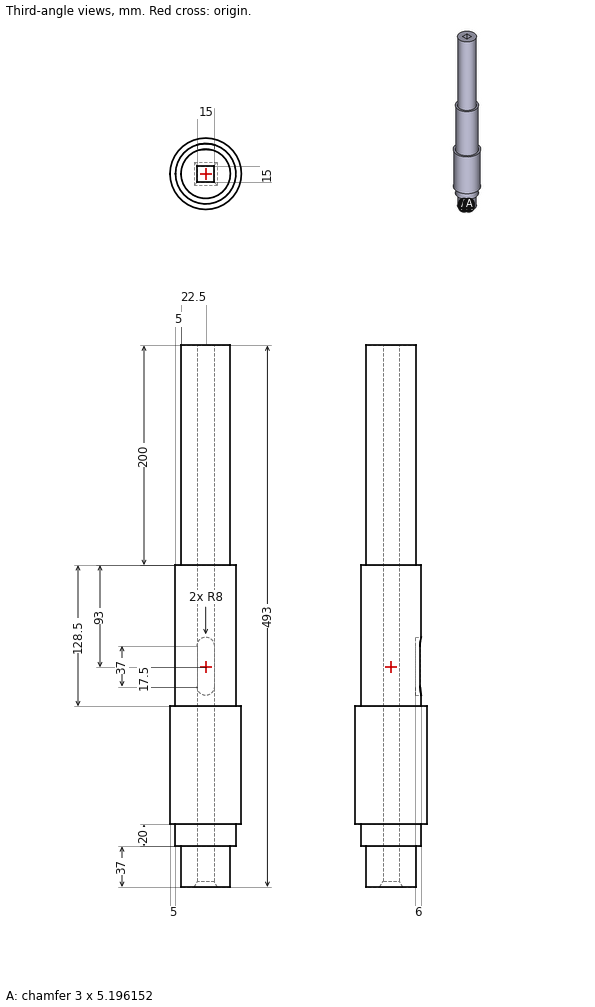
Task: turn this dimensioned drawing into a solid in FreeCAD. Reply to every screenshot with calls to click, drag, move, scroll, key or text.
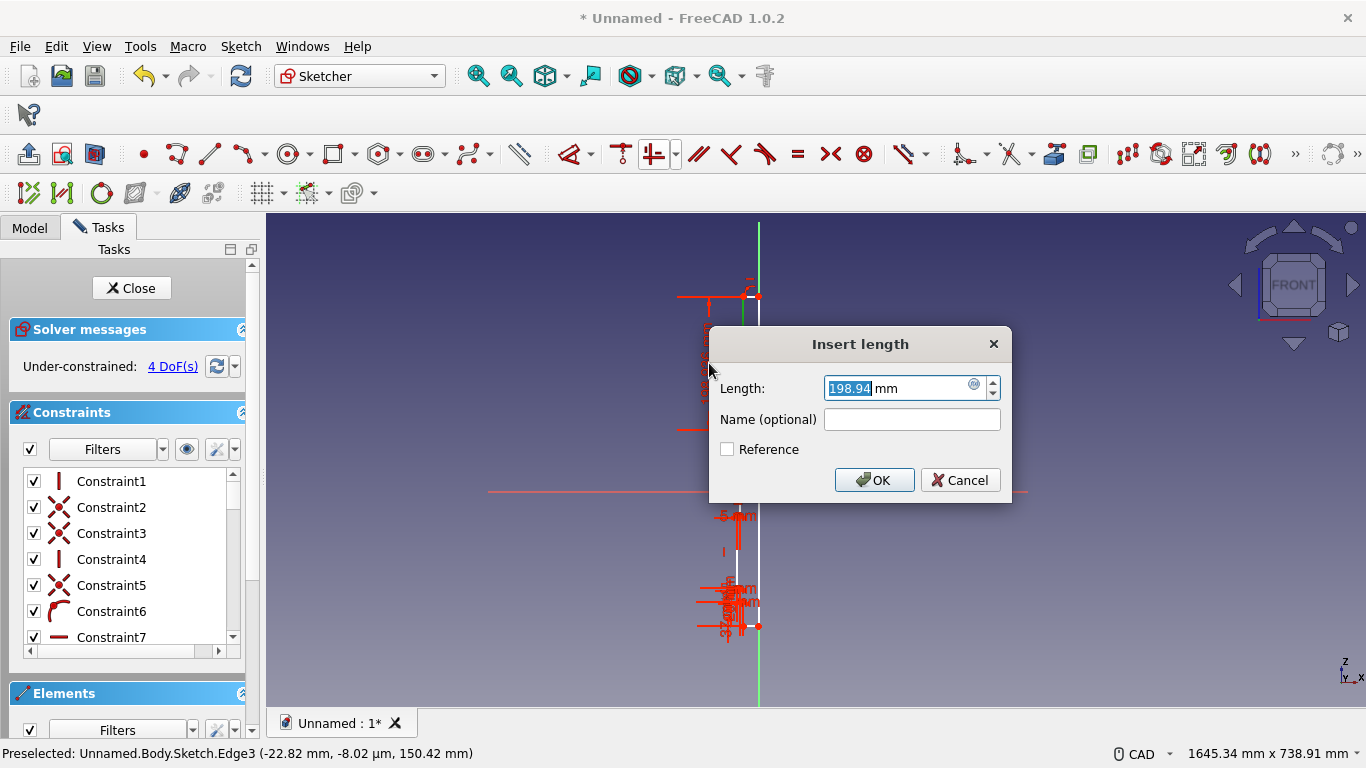
text(200)
key(Return)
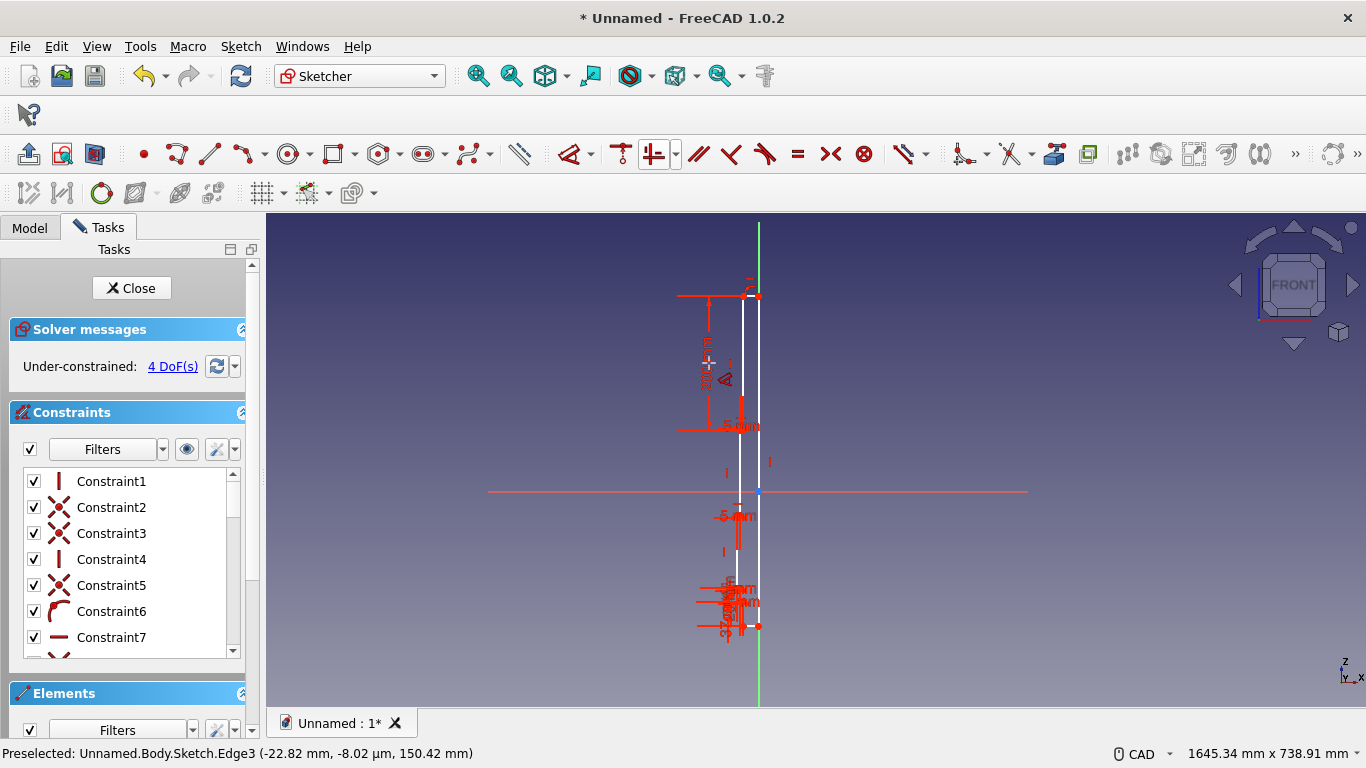
click(759, 395)
click(793, 461)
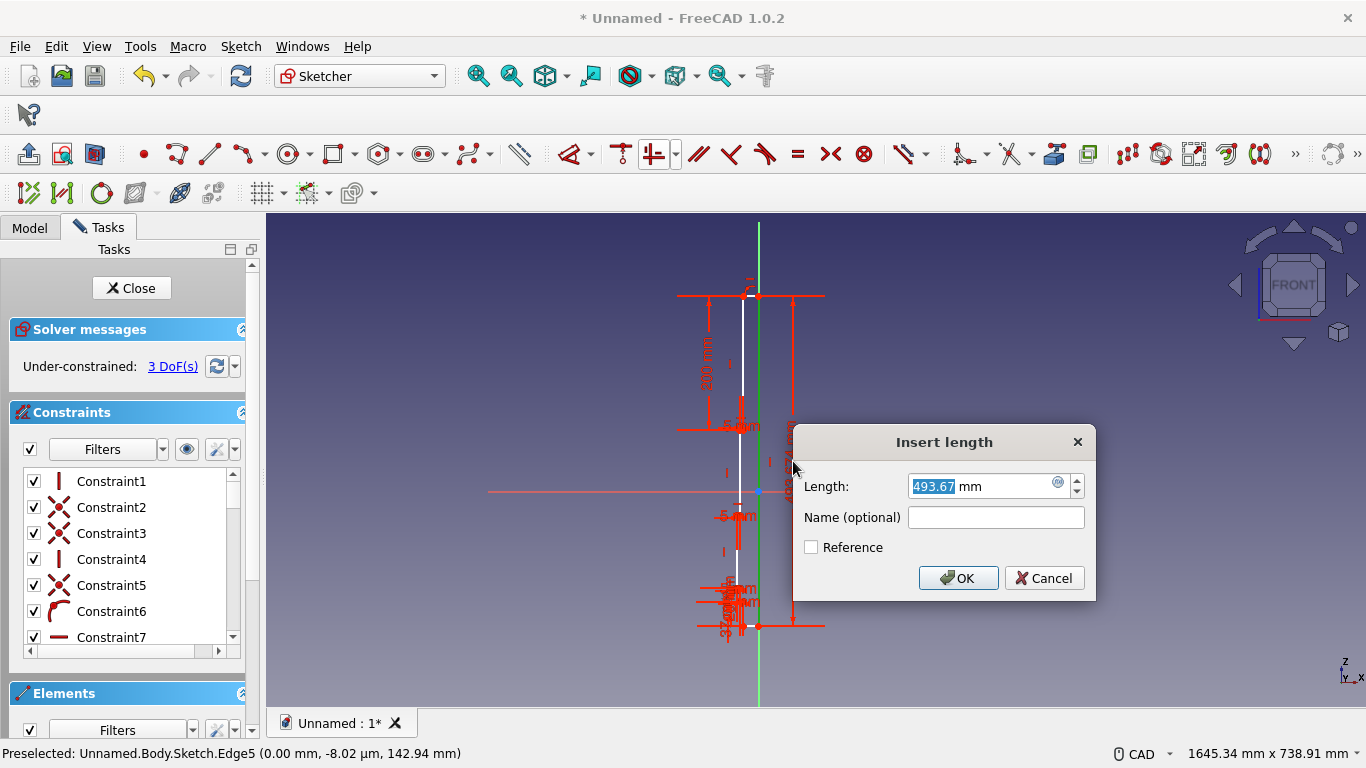
text(493)
key(Return)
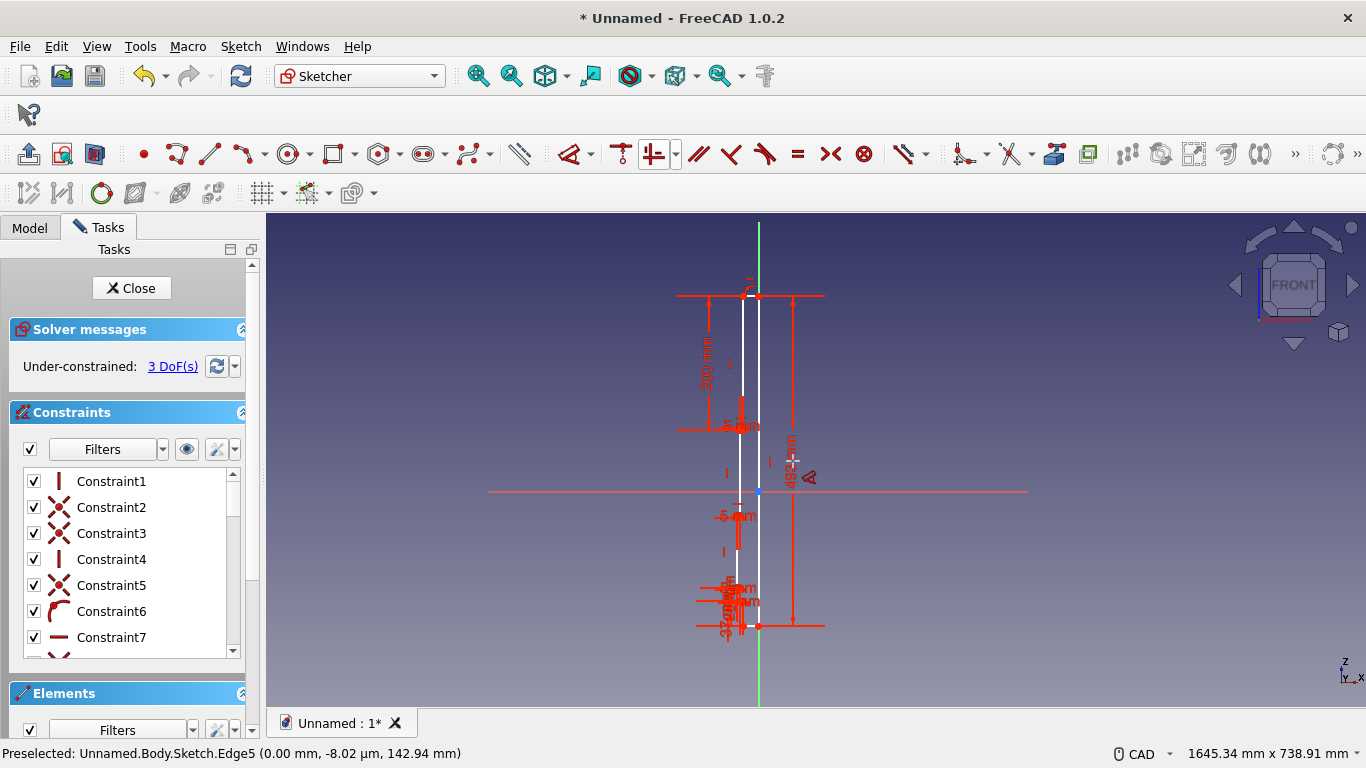
scroll(740, 430, up, 7)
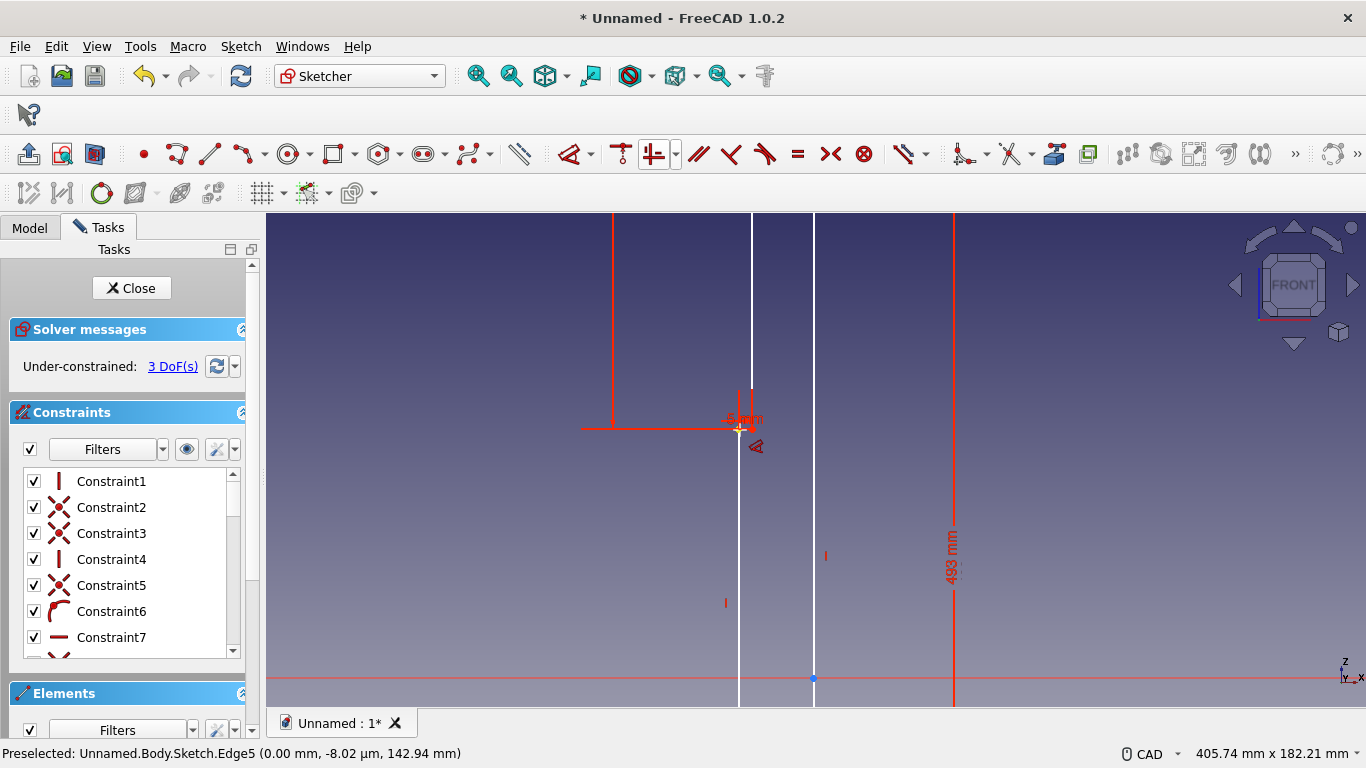
click(739, 429)
click(848, 554)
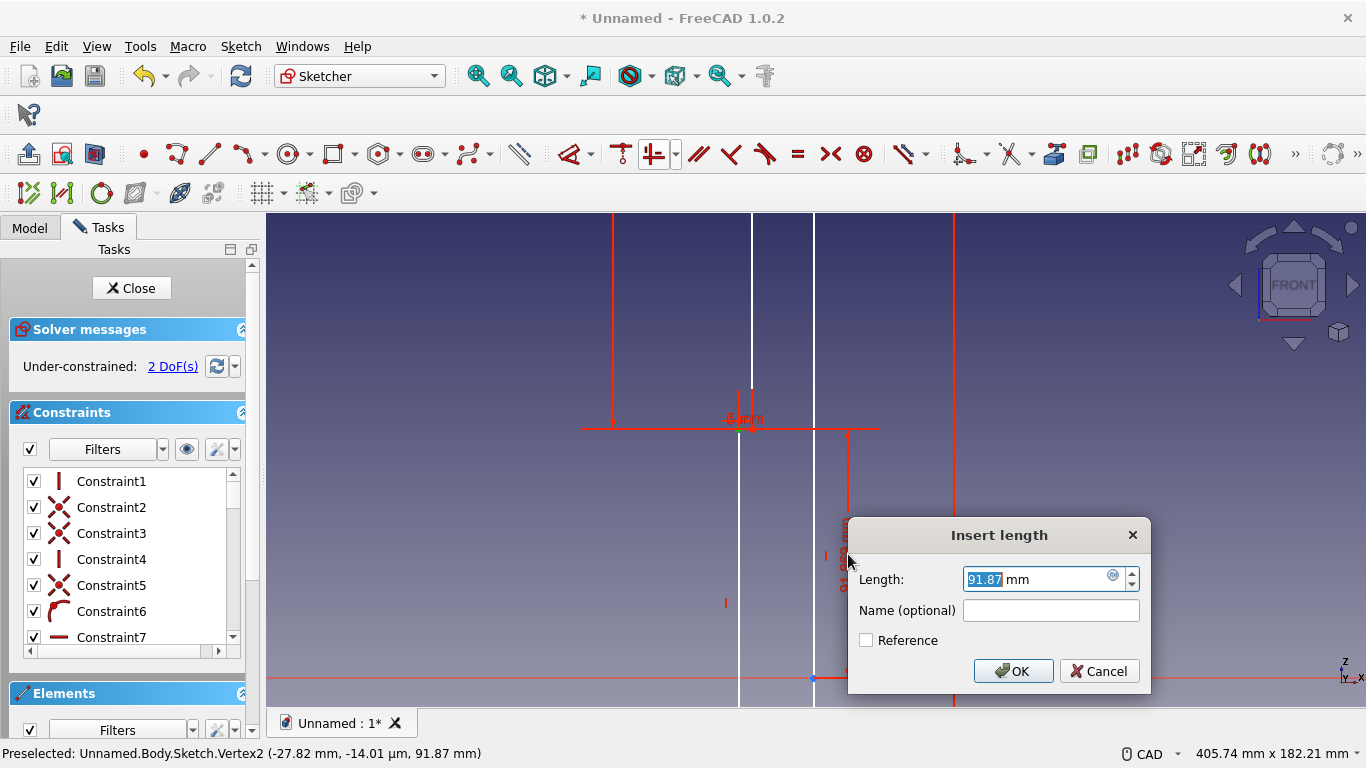
text(93)
key(Return)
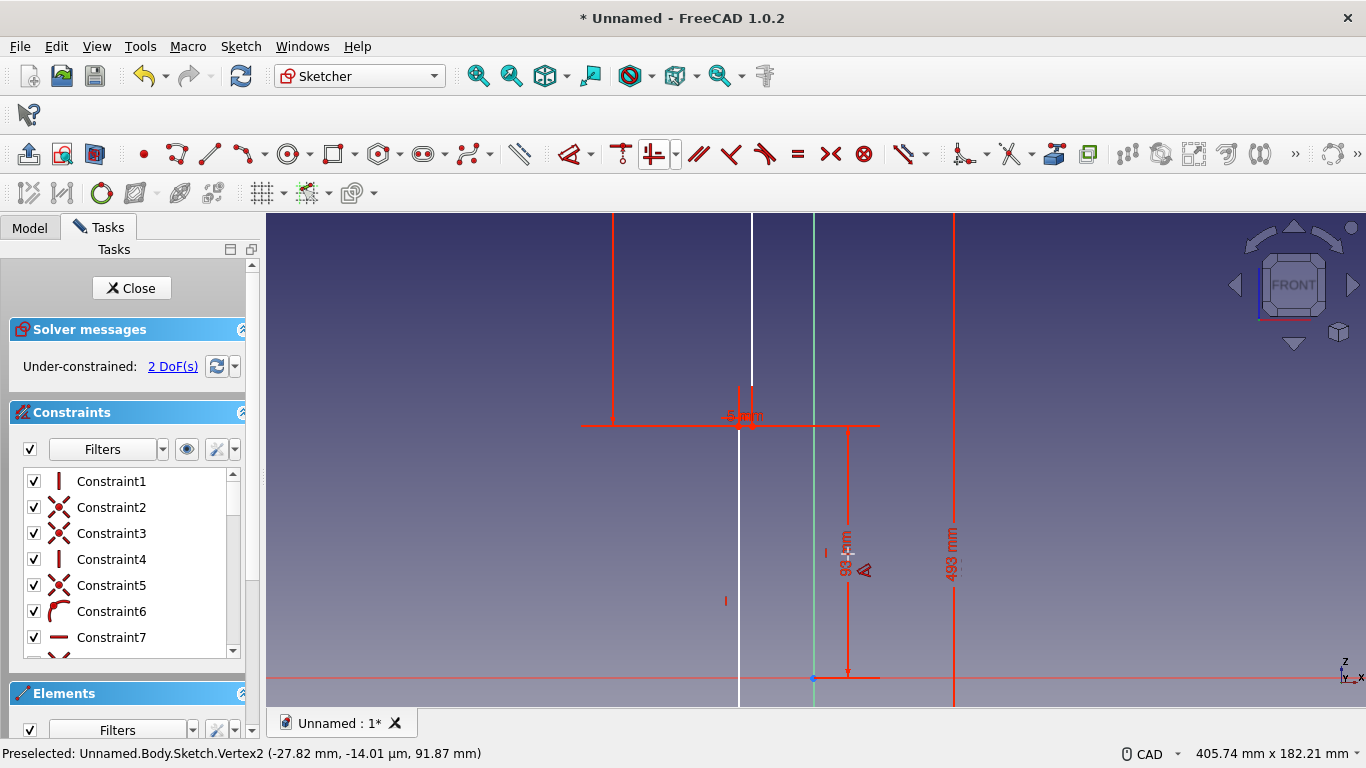
scroll(740, 430, down, 7)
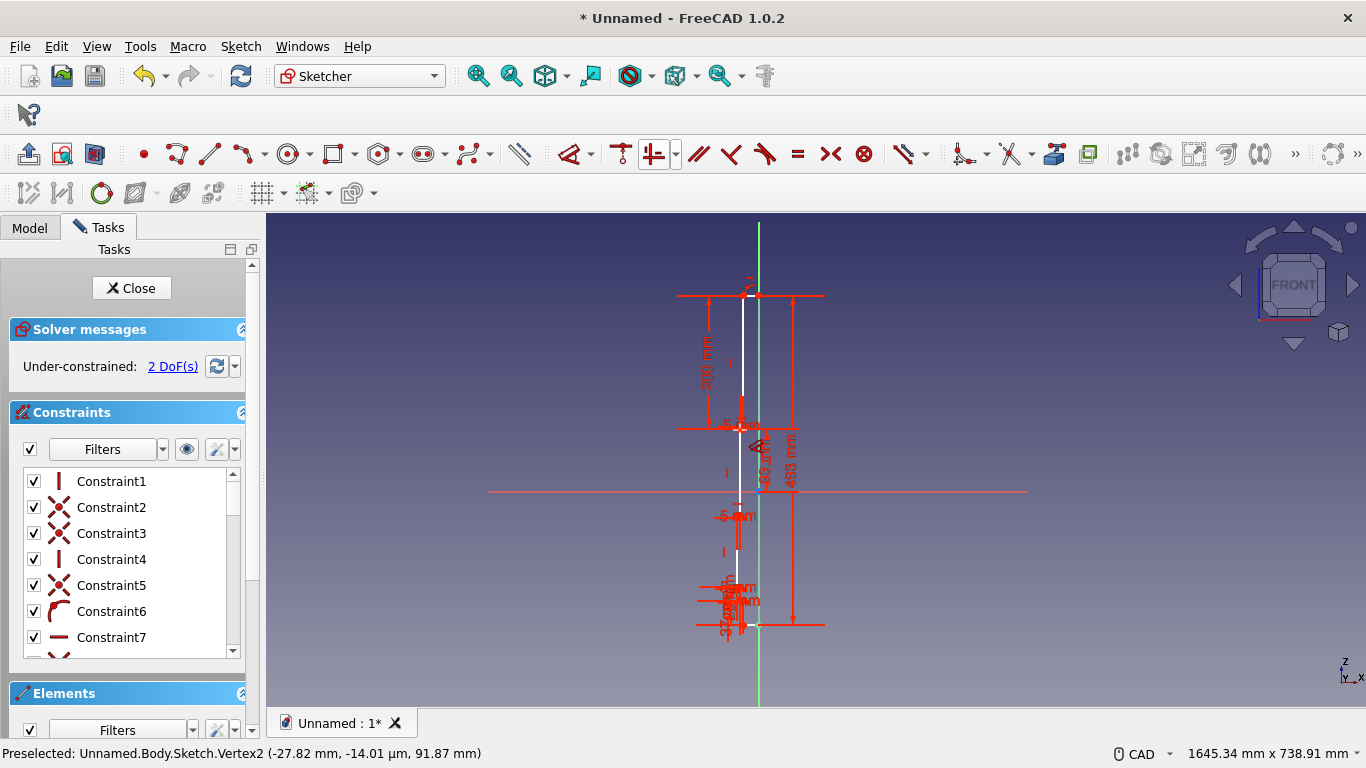
scroll(748, 296, up, 6)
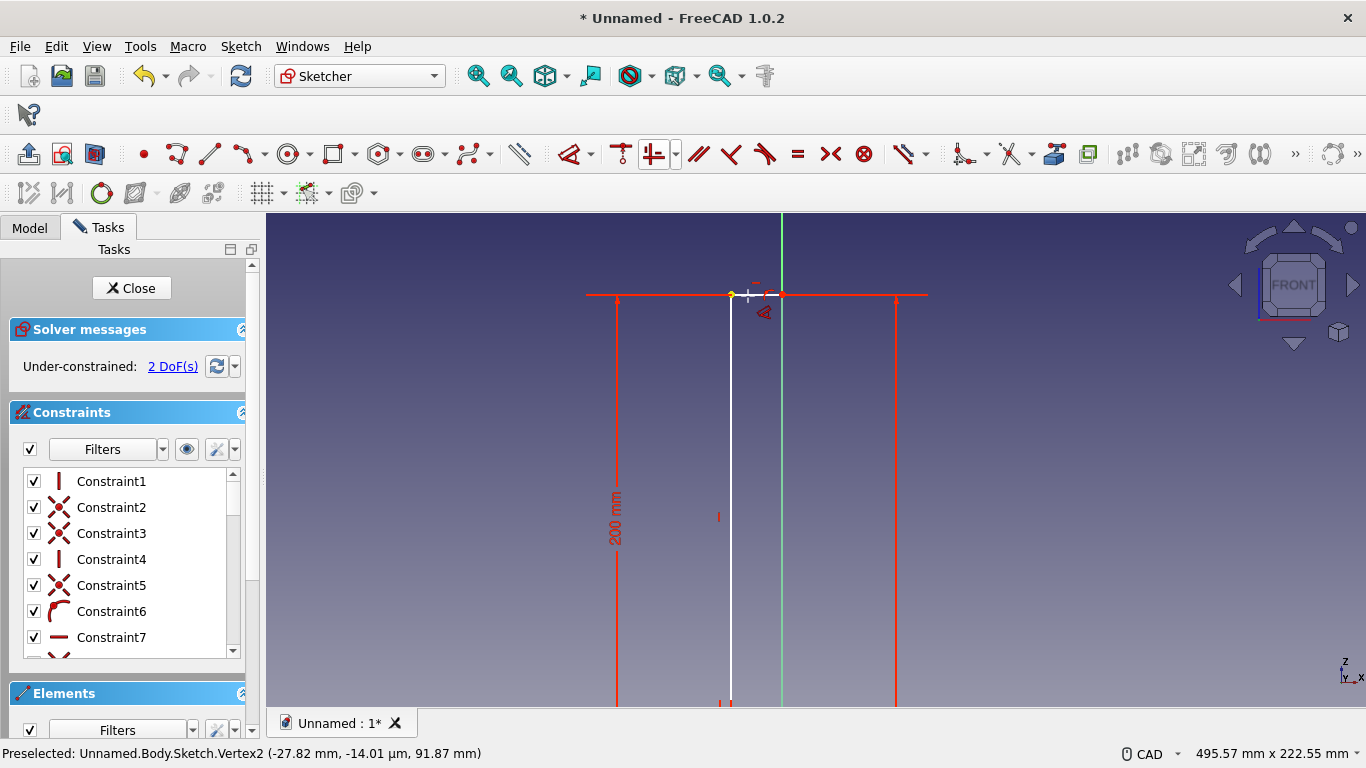
click(747, 295)
click(757, 261)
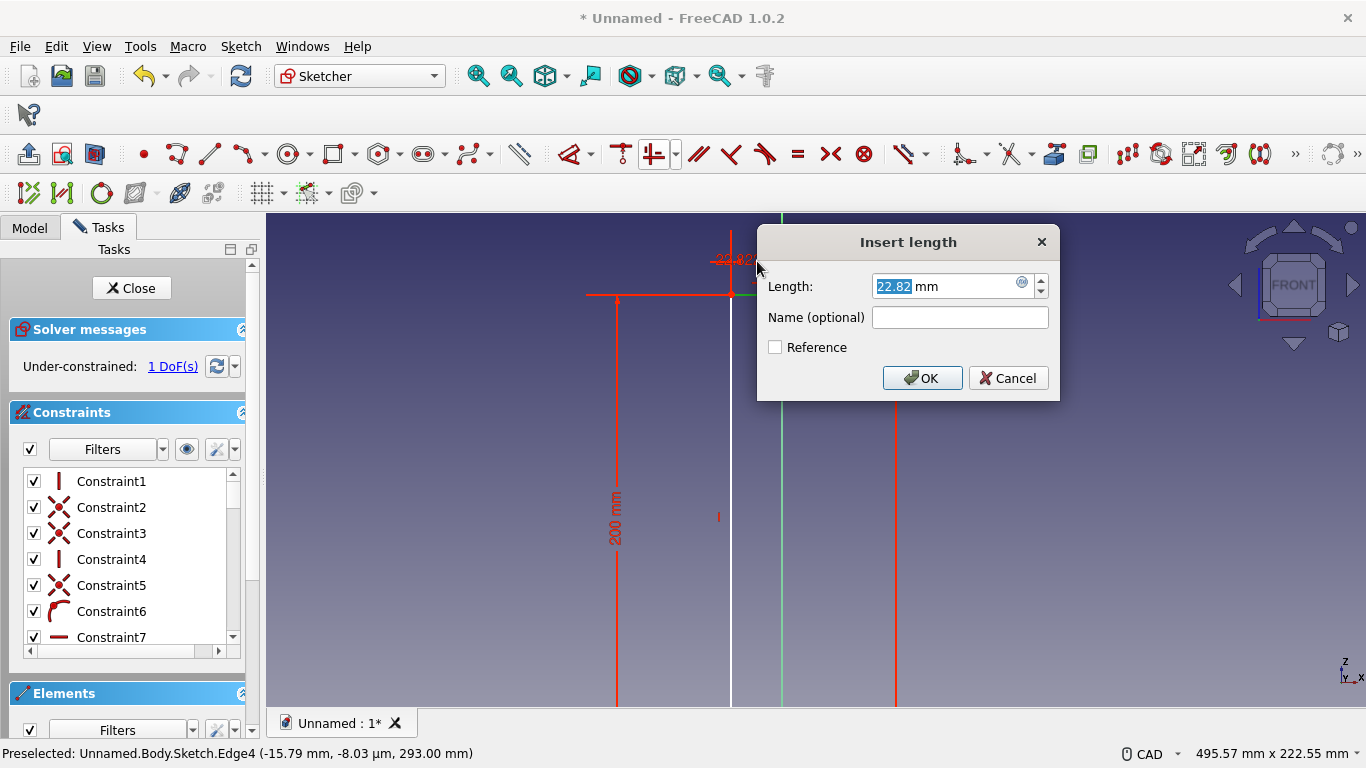
text(22.5)
key(Return)